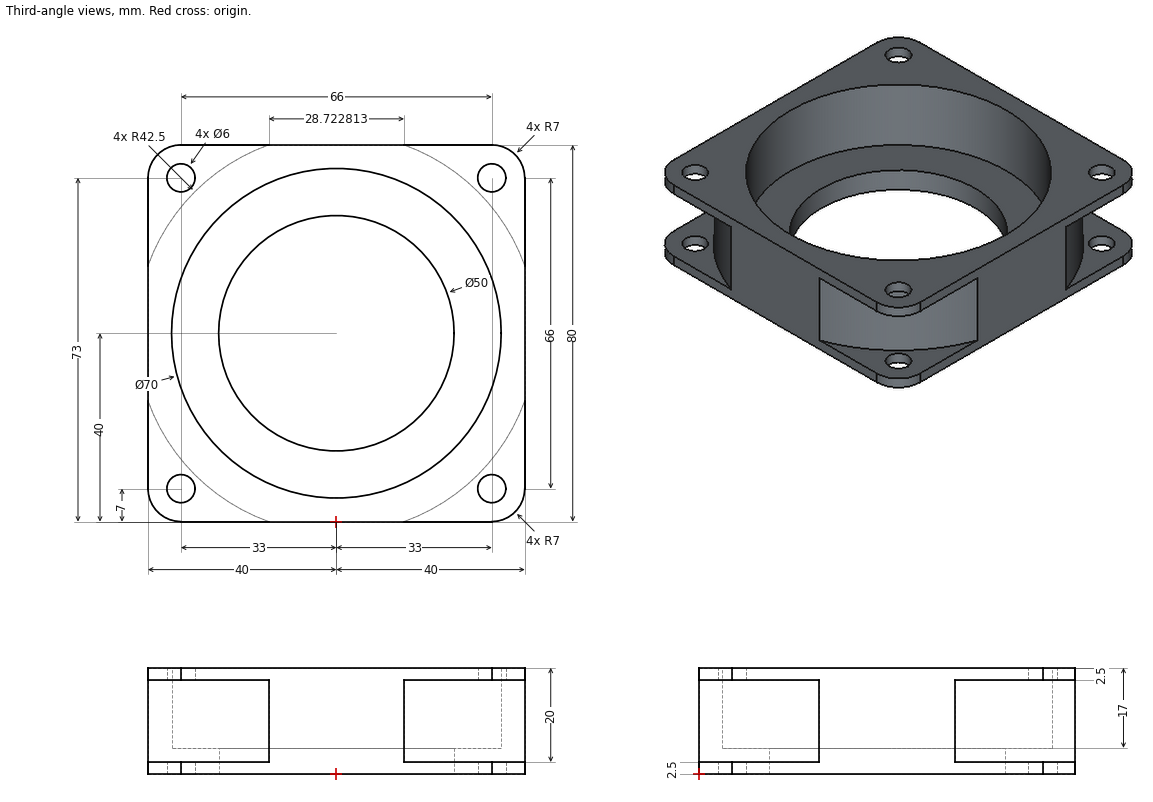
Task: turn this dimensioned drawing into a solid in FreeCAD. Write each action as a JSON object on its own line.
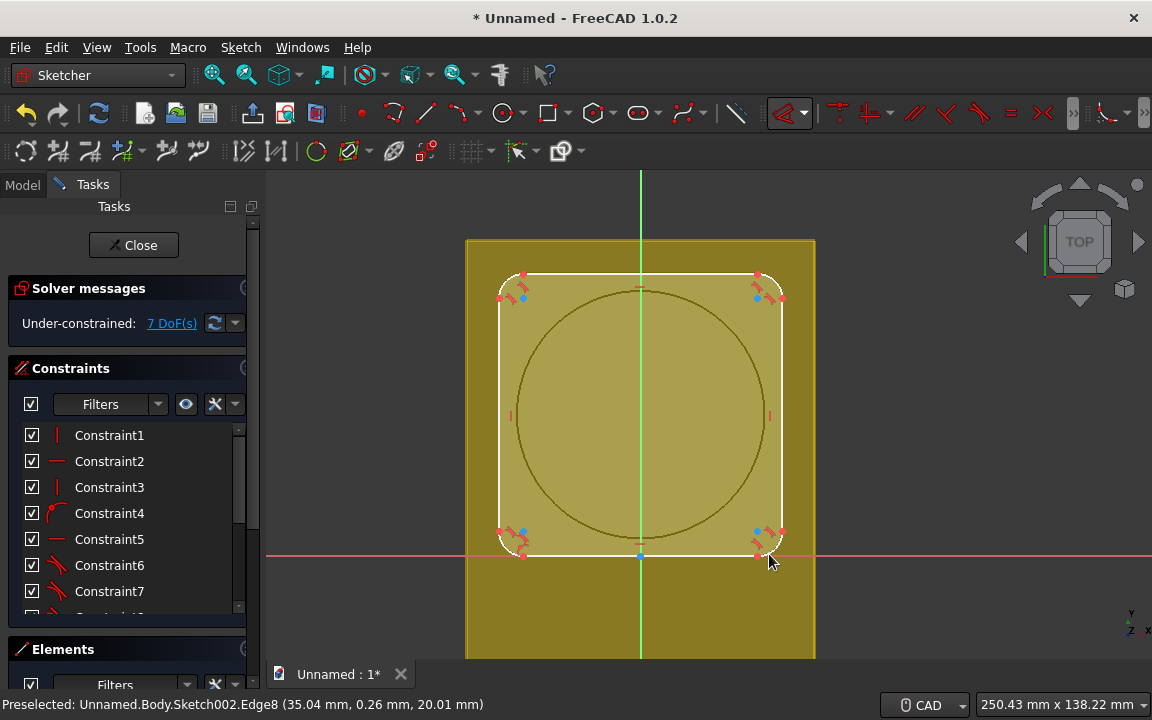
{"action": "left_click", "coordinate": [780, 288]}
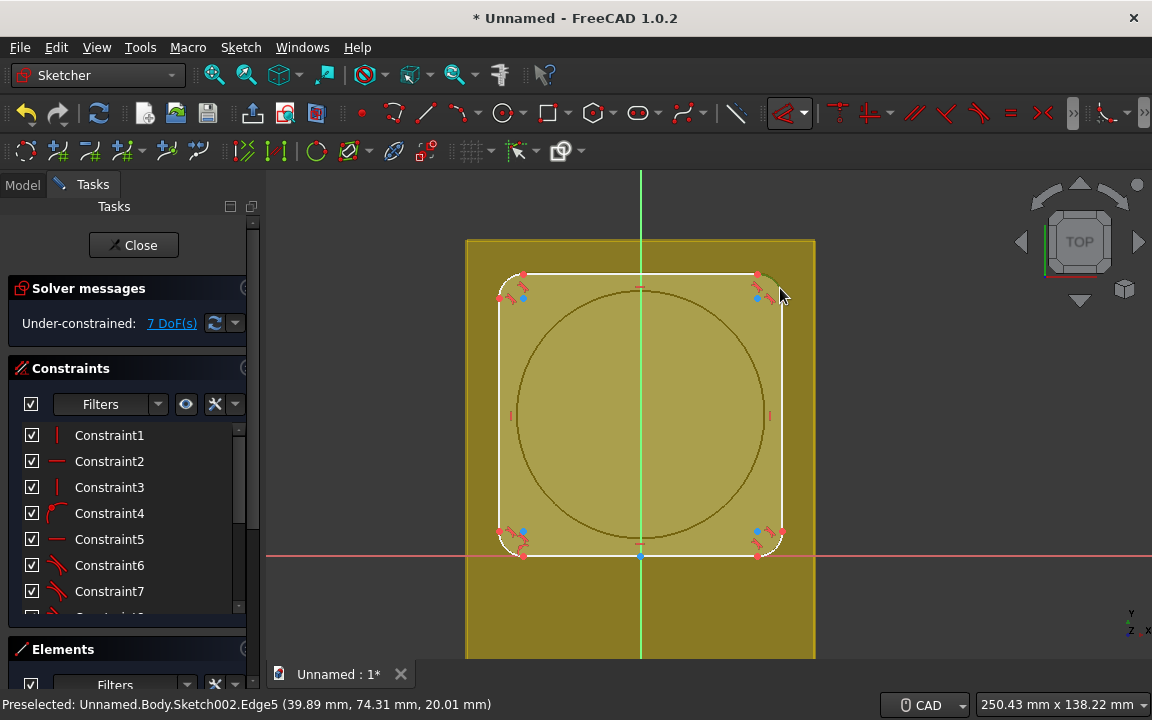
{"action": "left_click", "coordinate": [512, 277]}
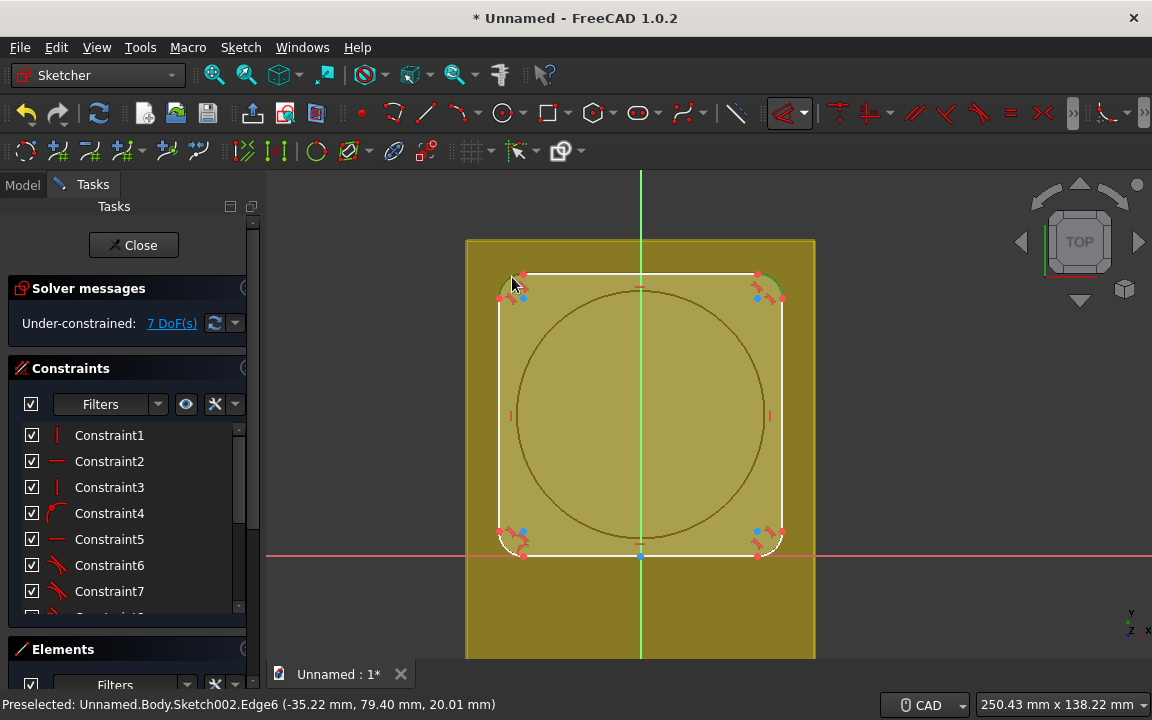
{"action": "left_click", "coordinate": [502, 543]}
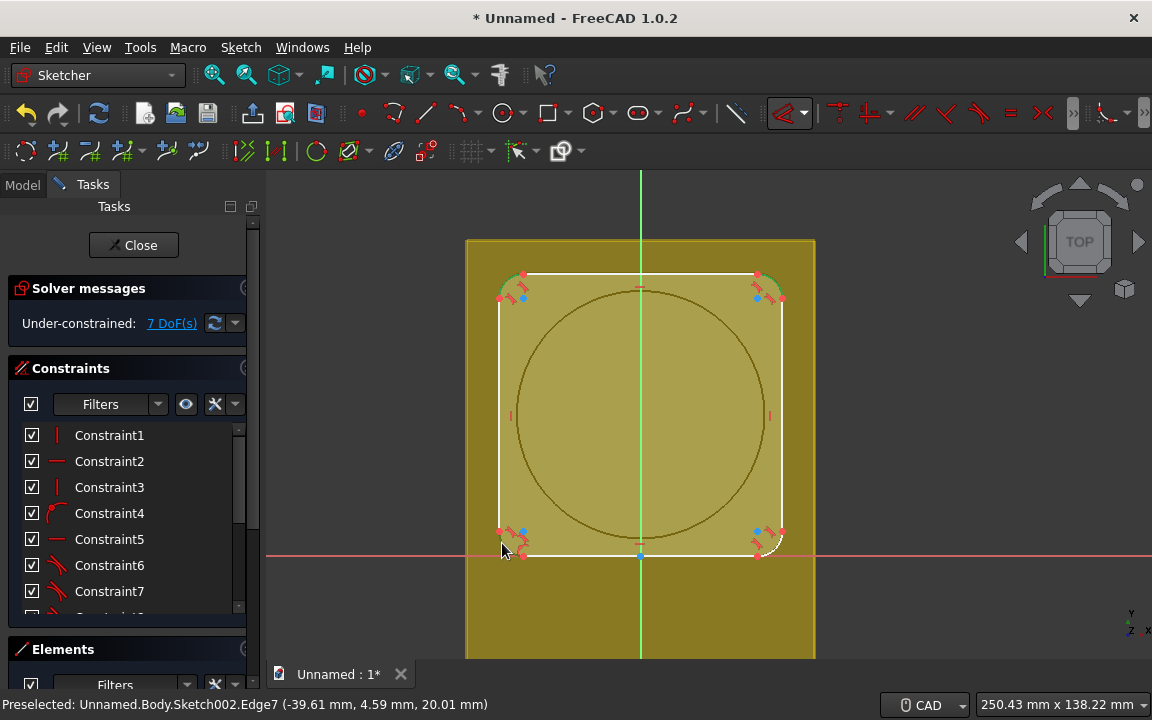
{"action": "left_click", "coordinate": [769, 554]}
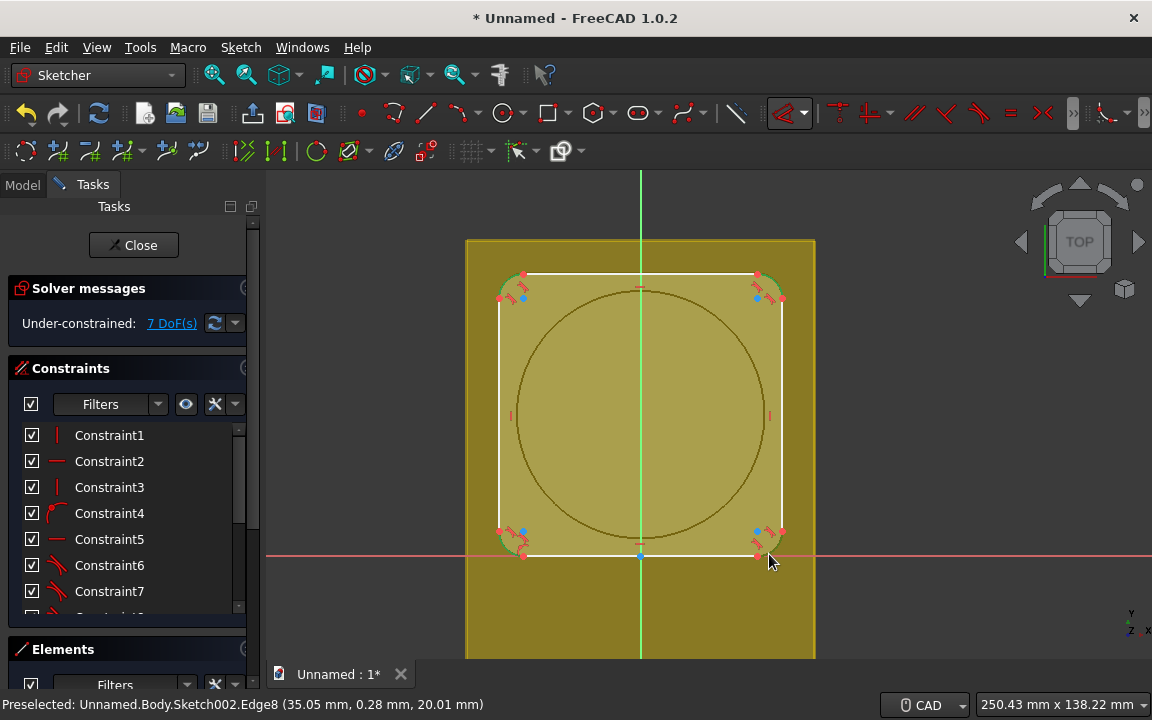
{"action": "key", "text": "e"}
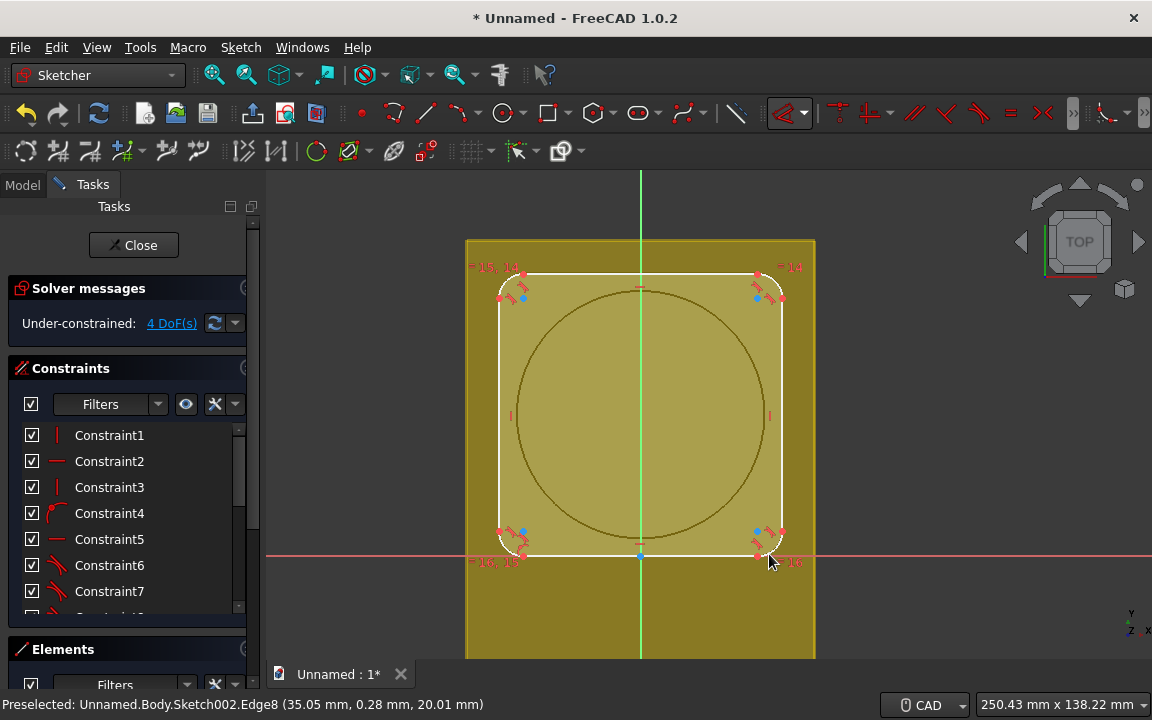
{"action": "key", "text": "d"}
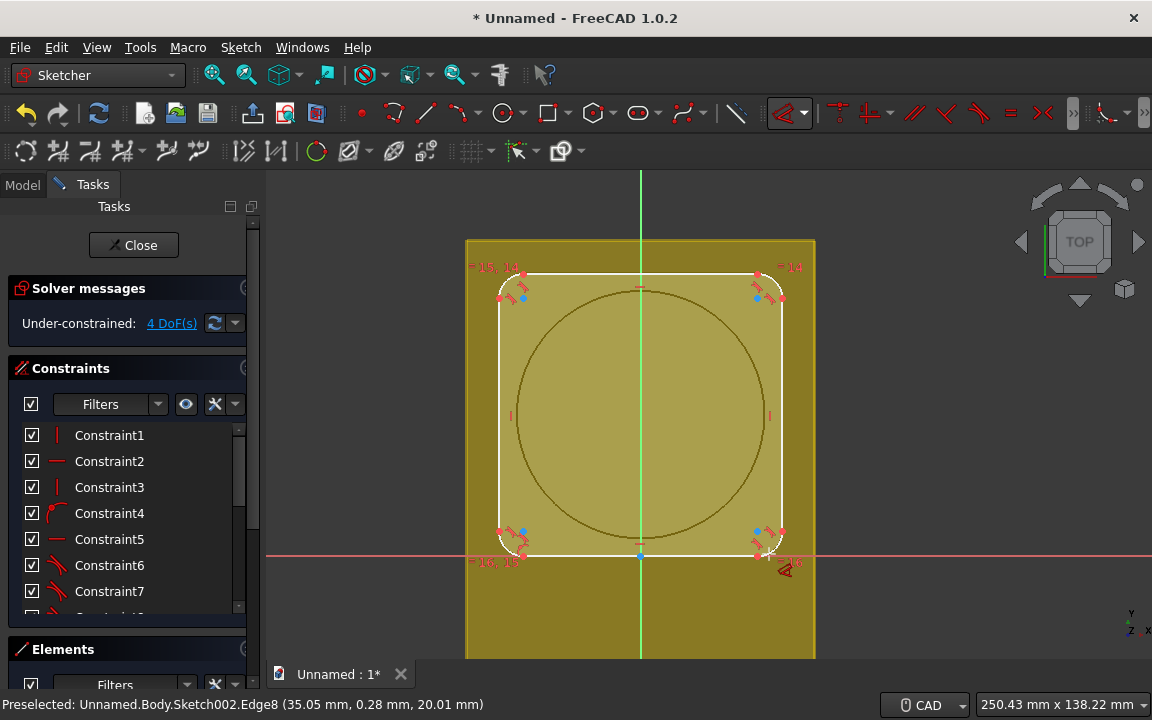
{"action": "scroll", "coordinate": [780, 288], "scroll_direction": "up", "scroll_amount": 3}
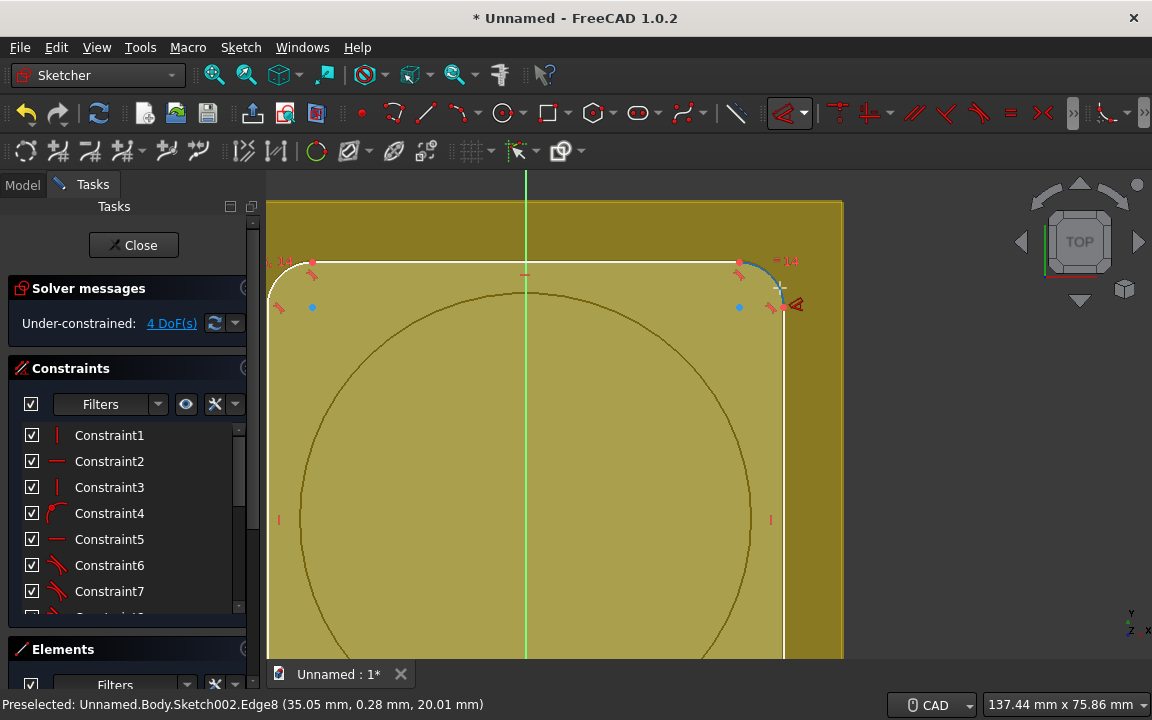
{"action": "left_click", "coordinate": [779, 287]}
{"action": "left_click", "coordinate": [808, 273]}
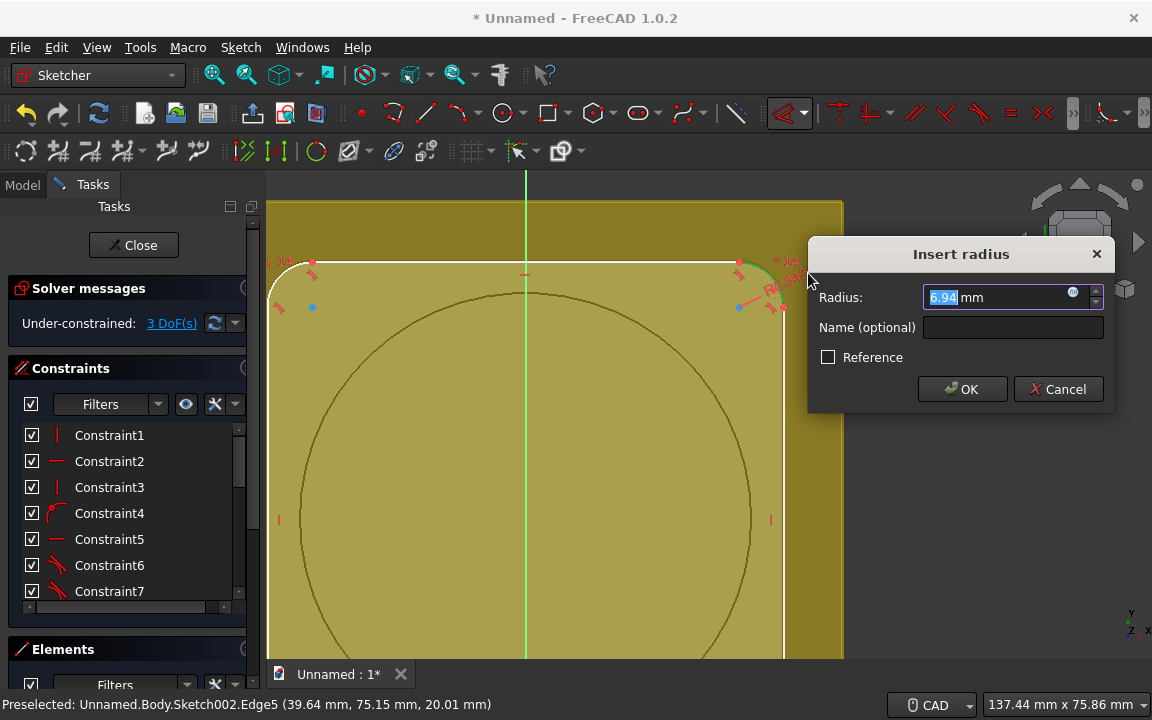
{"action": "type", "text": "7"}
{"action": "key", "text": "Return"}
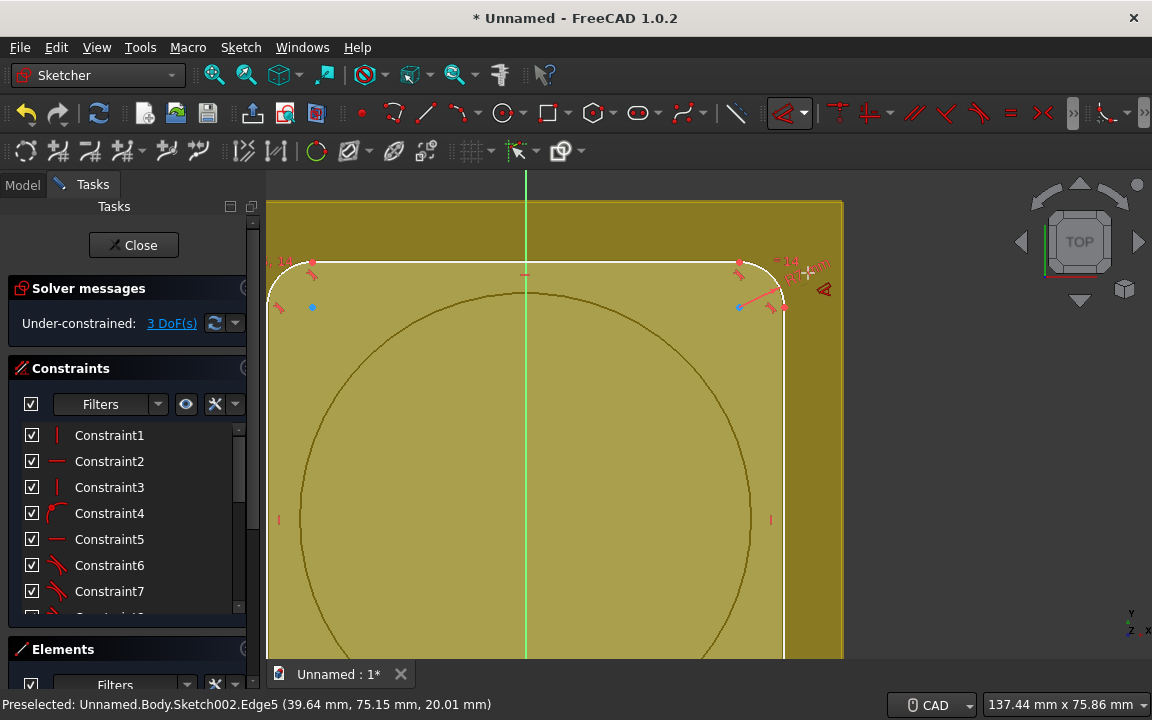
{"action": "left_click", "coordinate": [784, 604]}
{"action": "left_click", "coordinate": [818, 469]}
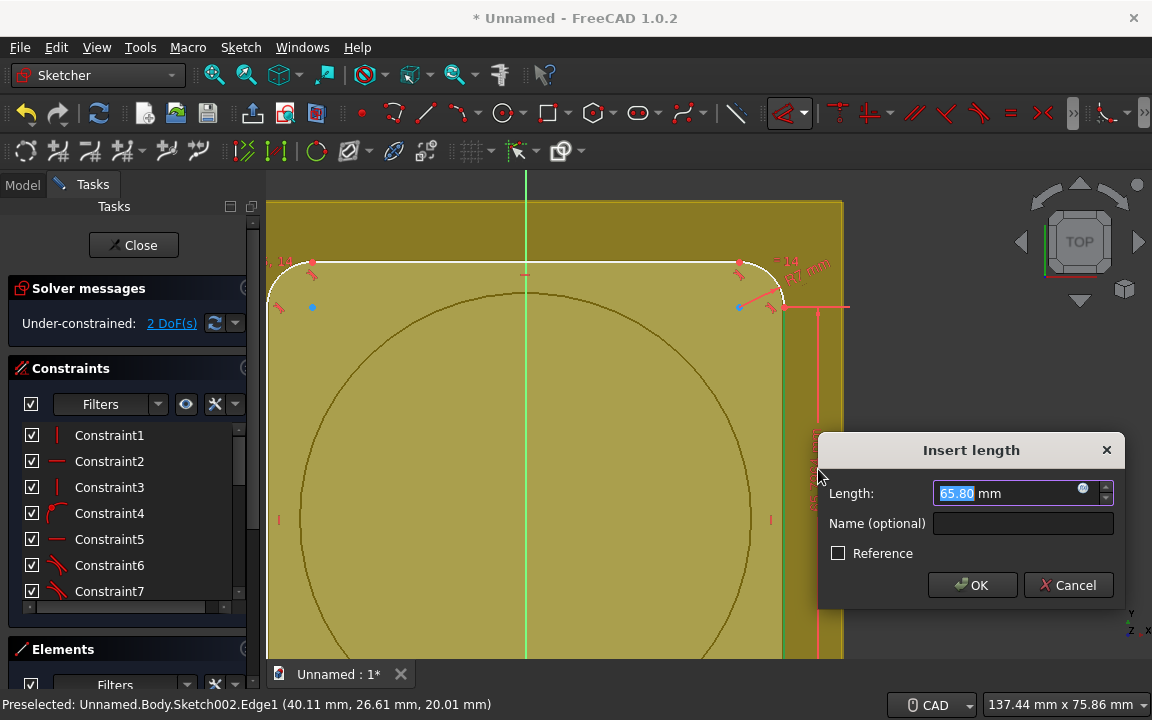
{"action": "type", "text": "66"}
{"action": "key", "text": "Return"}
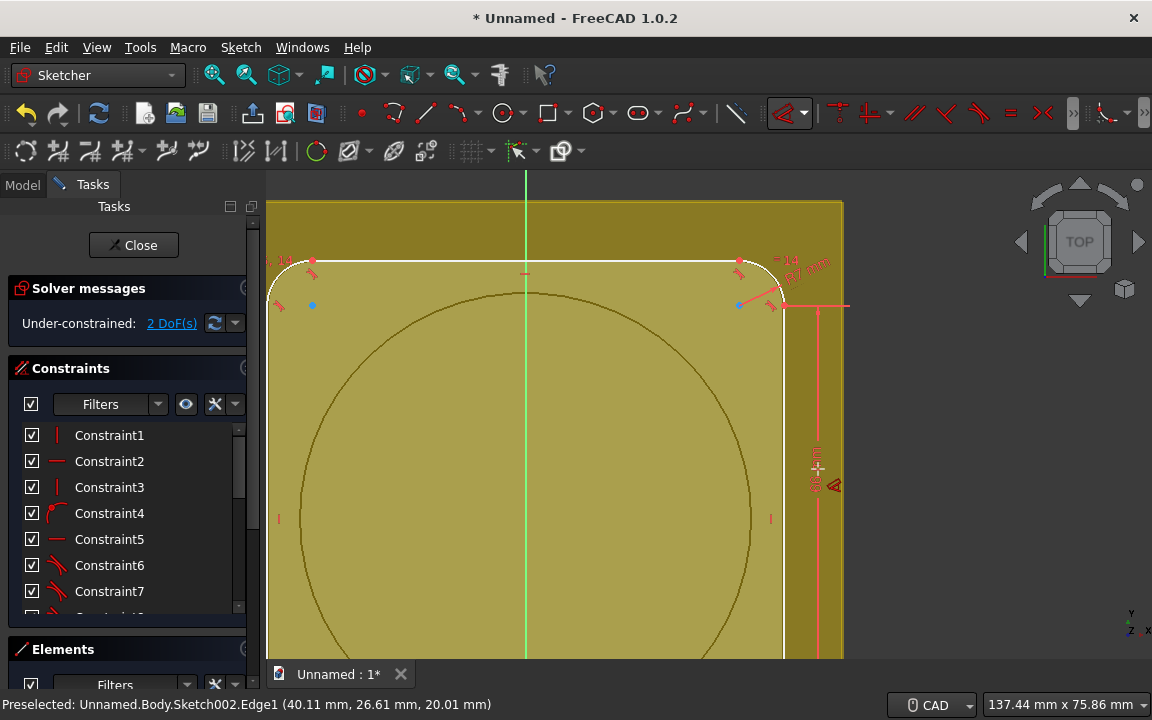
{"action": "left_click", "coordinate": [611, 261]}
{"action": "left_click", "coordinate": [428, 227]}